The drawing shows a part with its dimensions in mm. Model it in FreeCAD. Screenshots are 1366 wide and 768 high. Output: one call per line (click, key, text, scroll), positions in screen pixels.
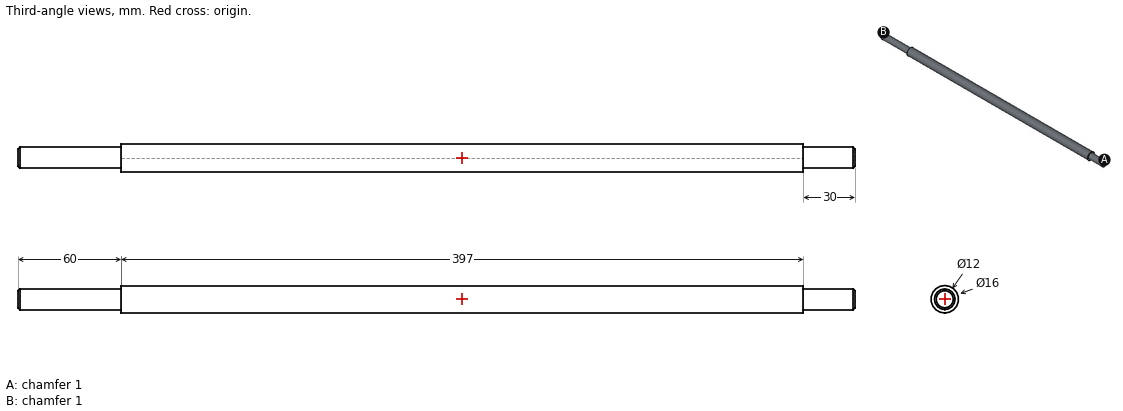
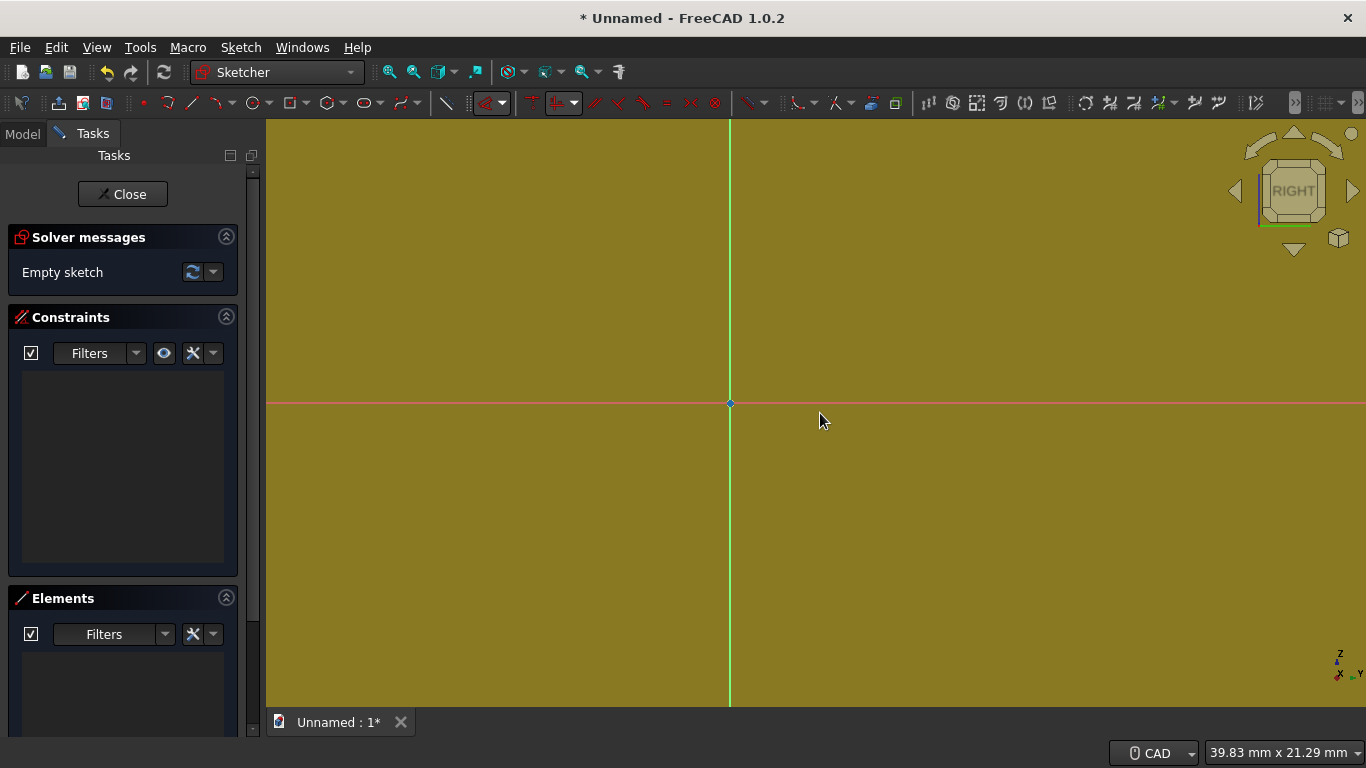
click(254, 104)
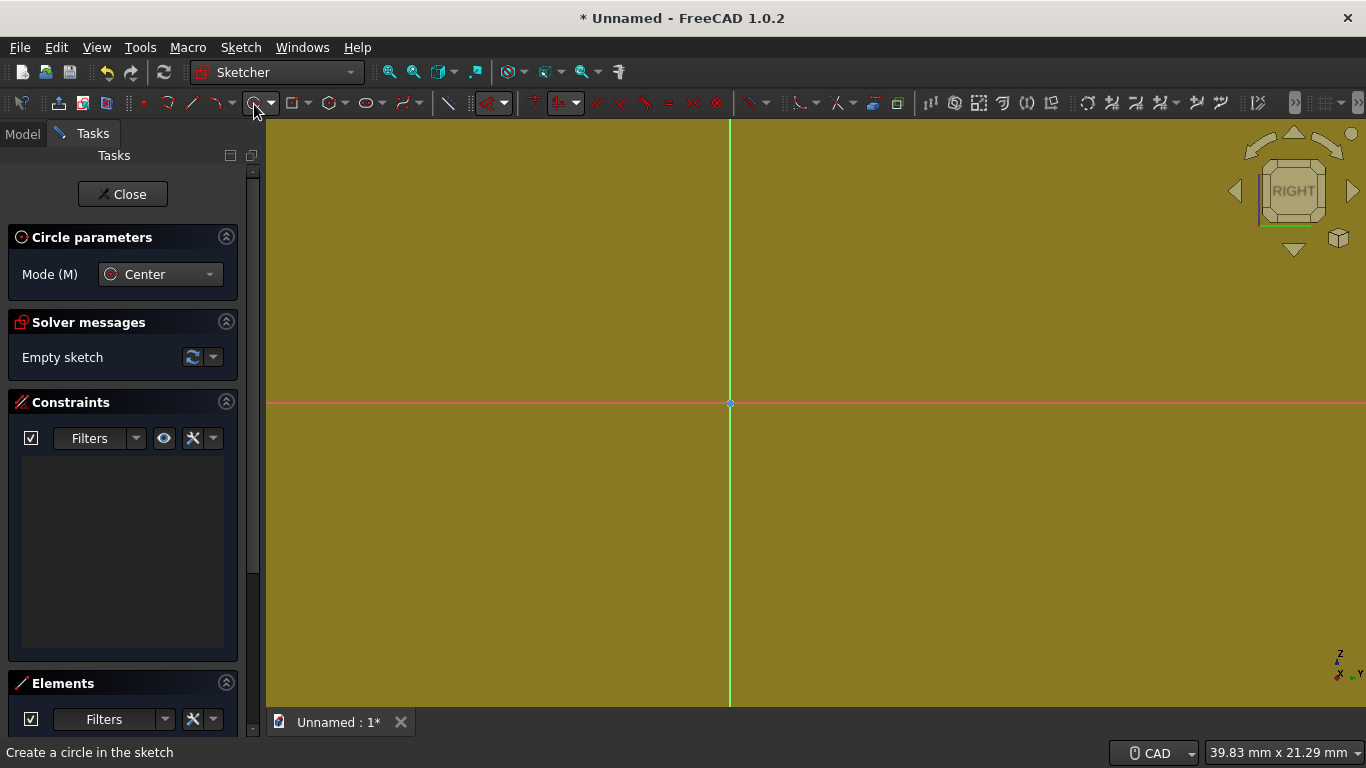
click(730, 403)
move(847, 286)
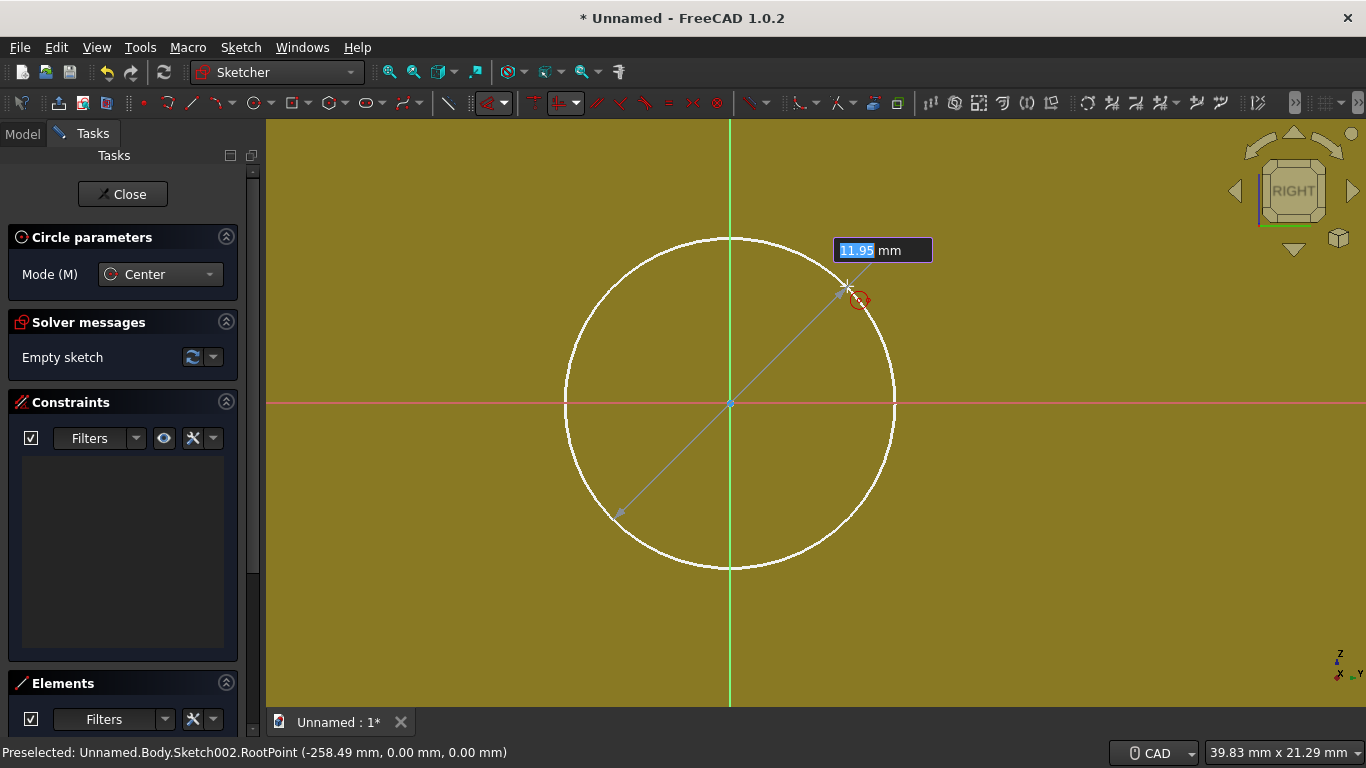
text(12)
key(Return)
key(Escape)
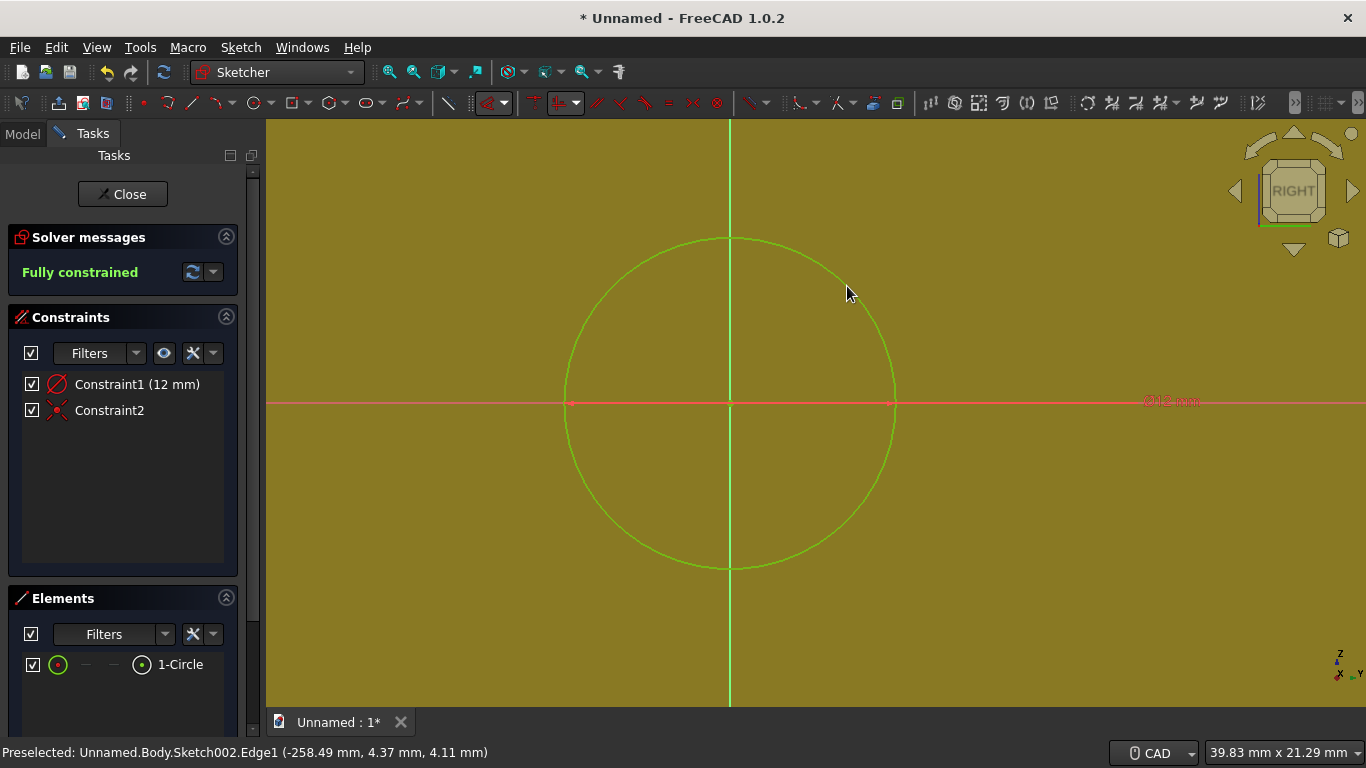
click(123, 194)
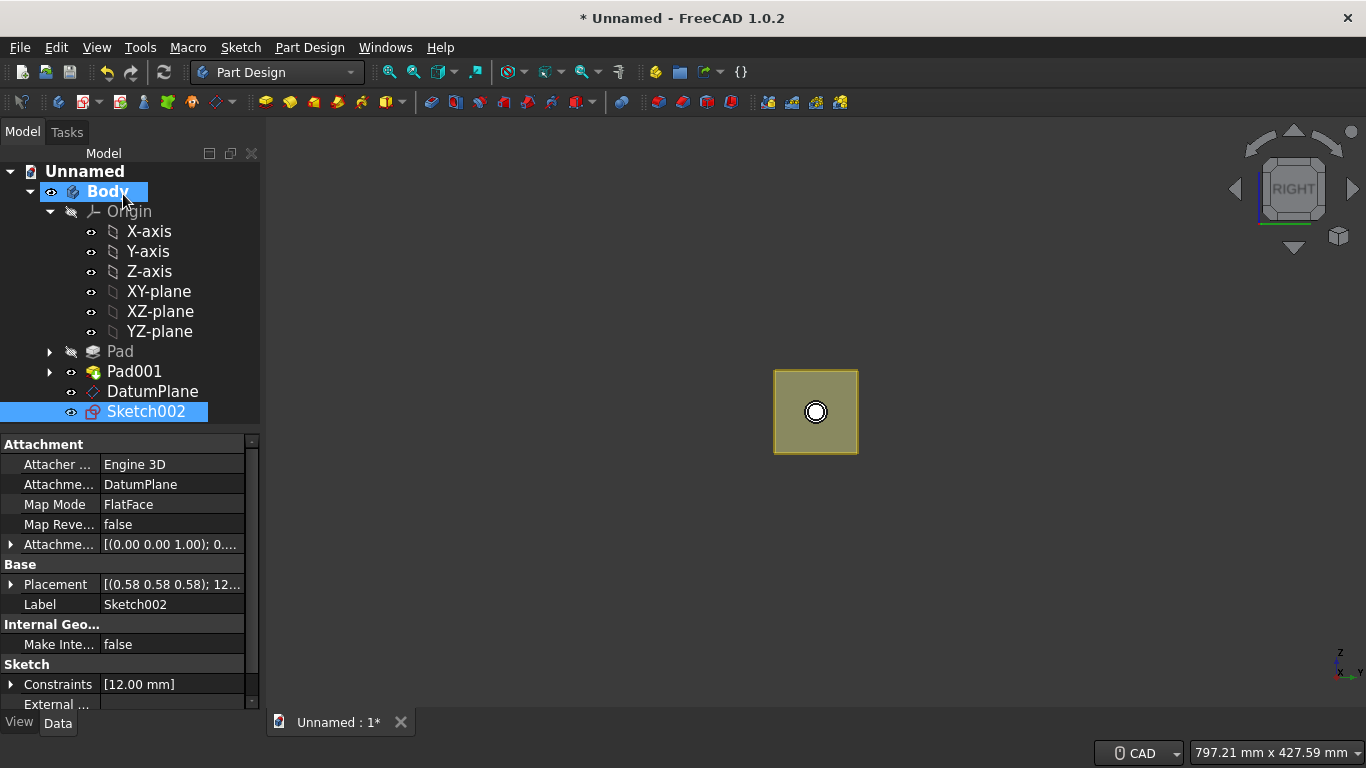
click(266, 102)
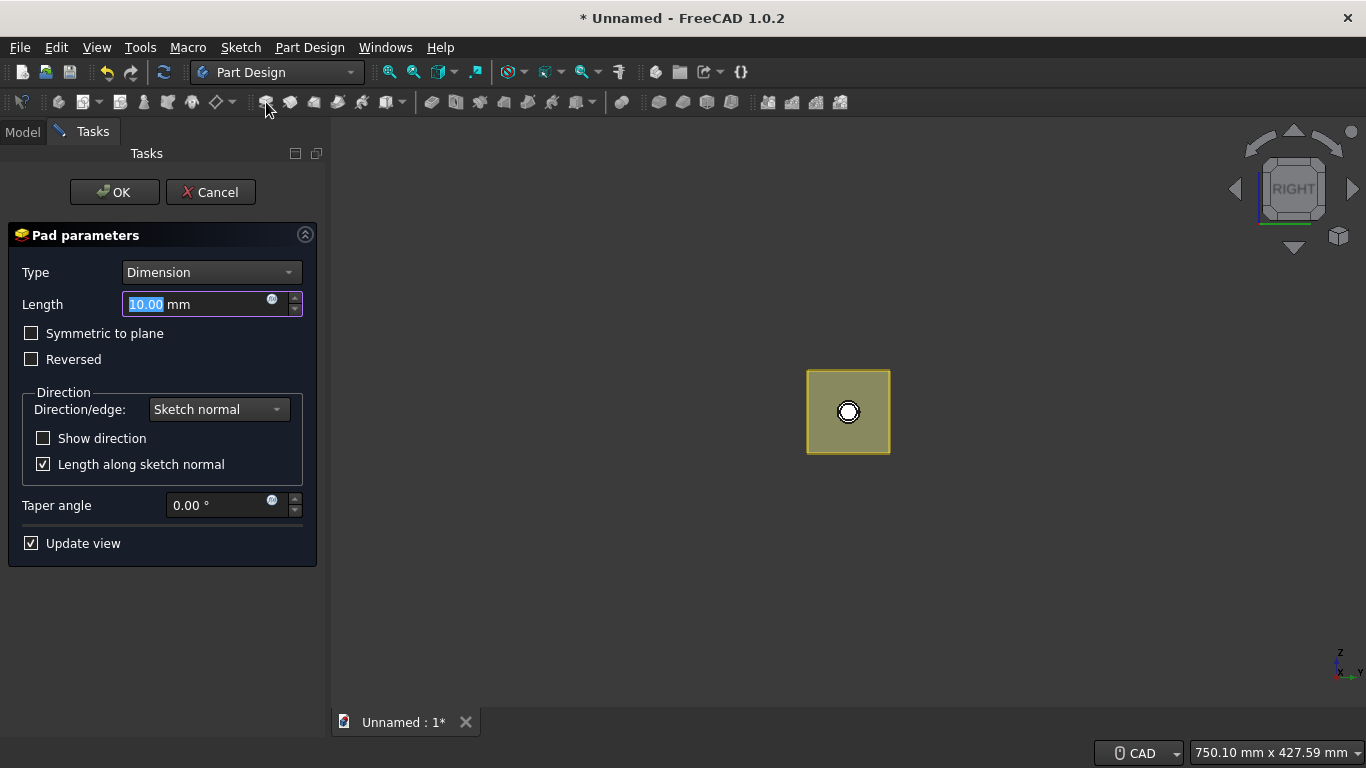
text(60)
key(Tab)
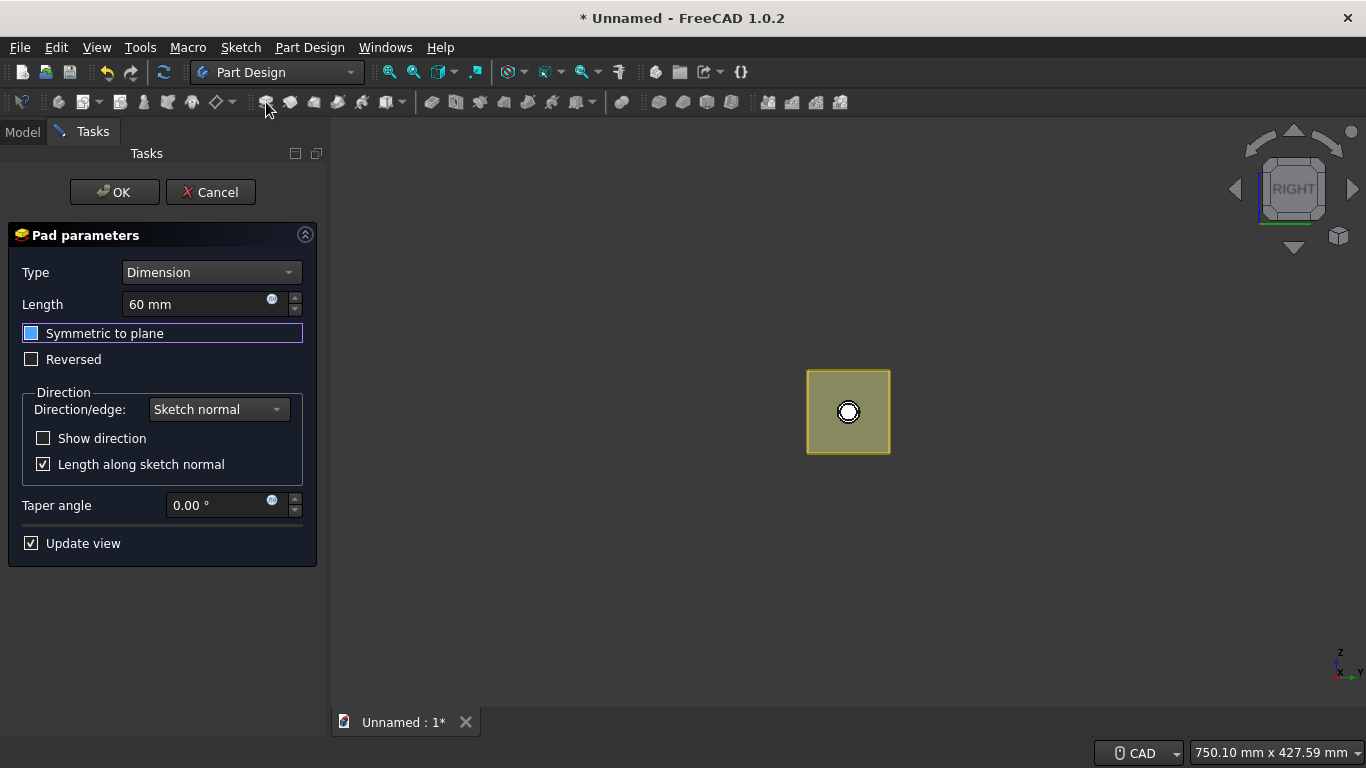
click(115, 192)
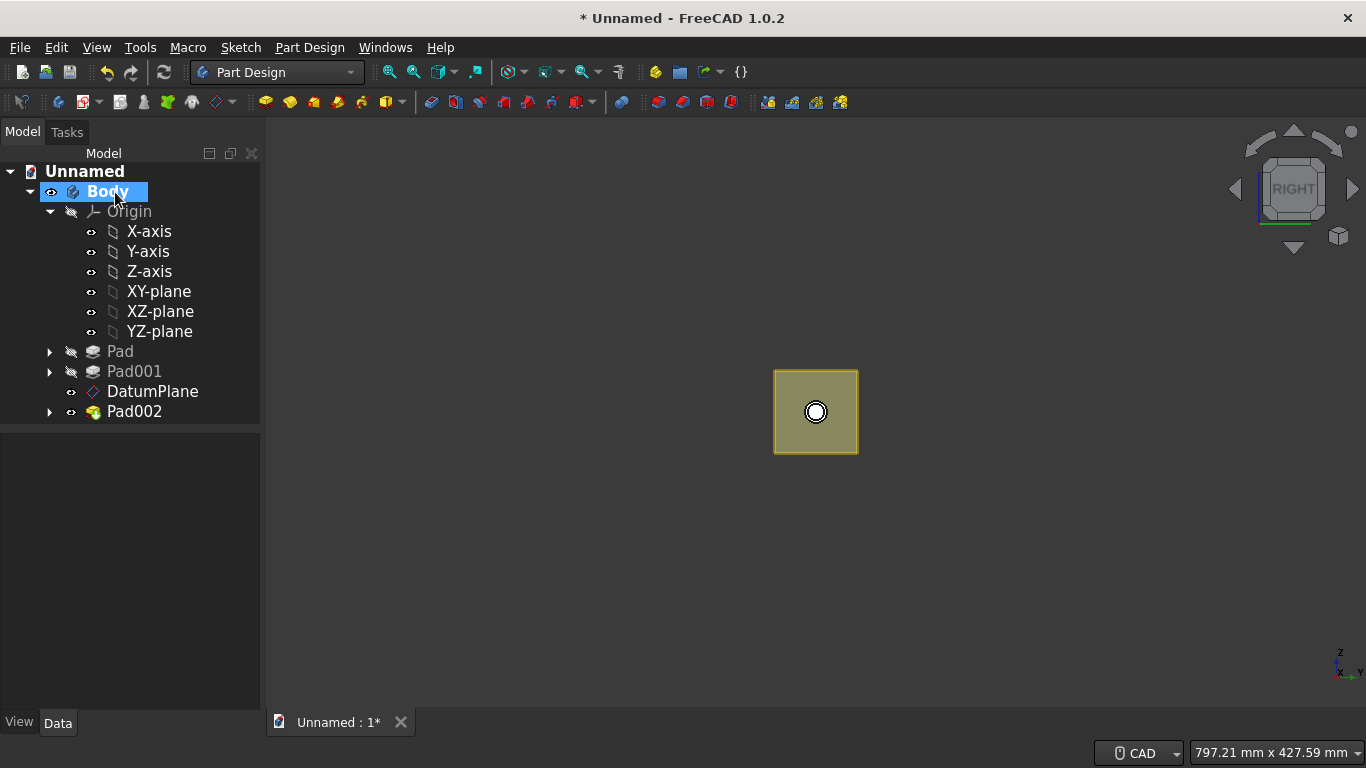
click(116, 392)
key(space)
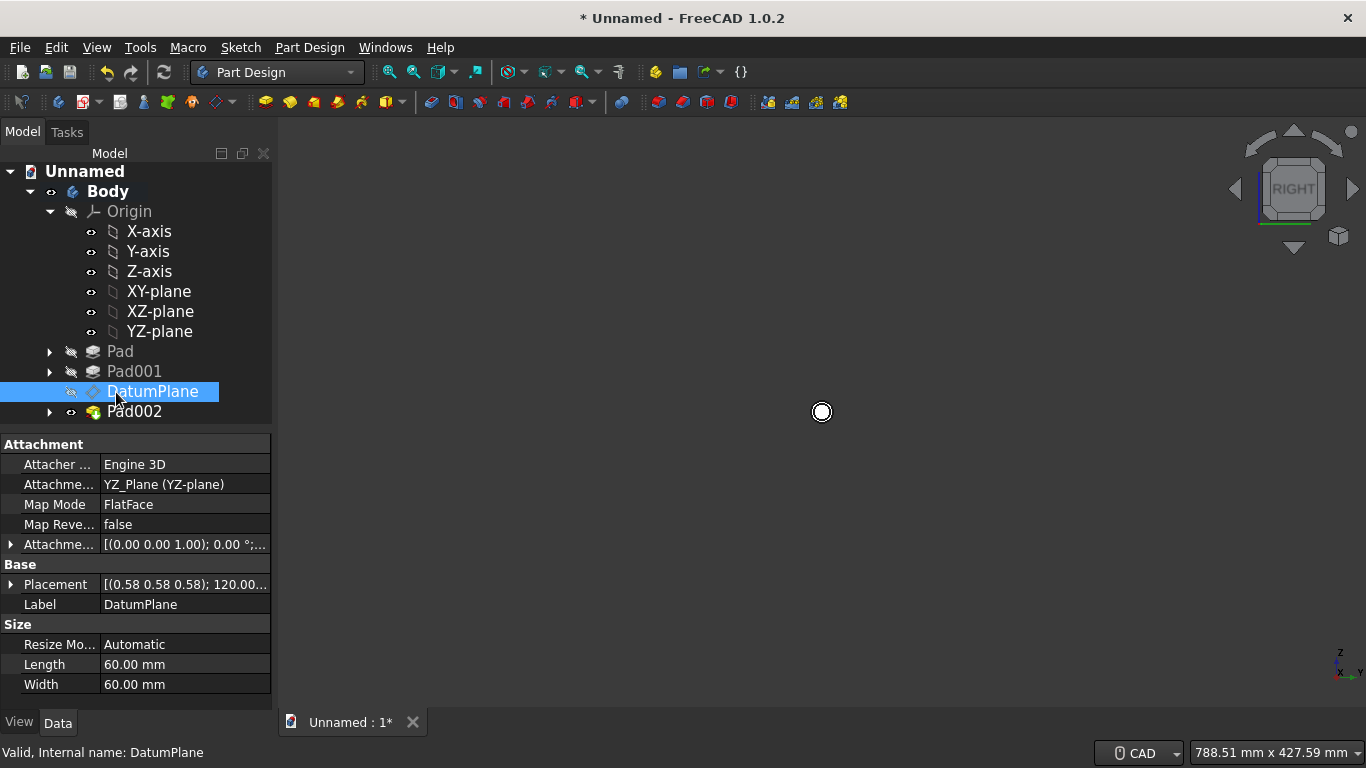
click(390, 72)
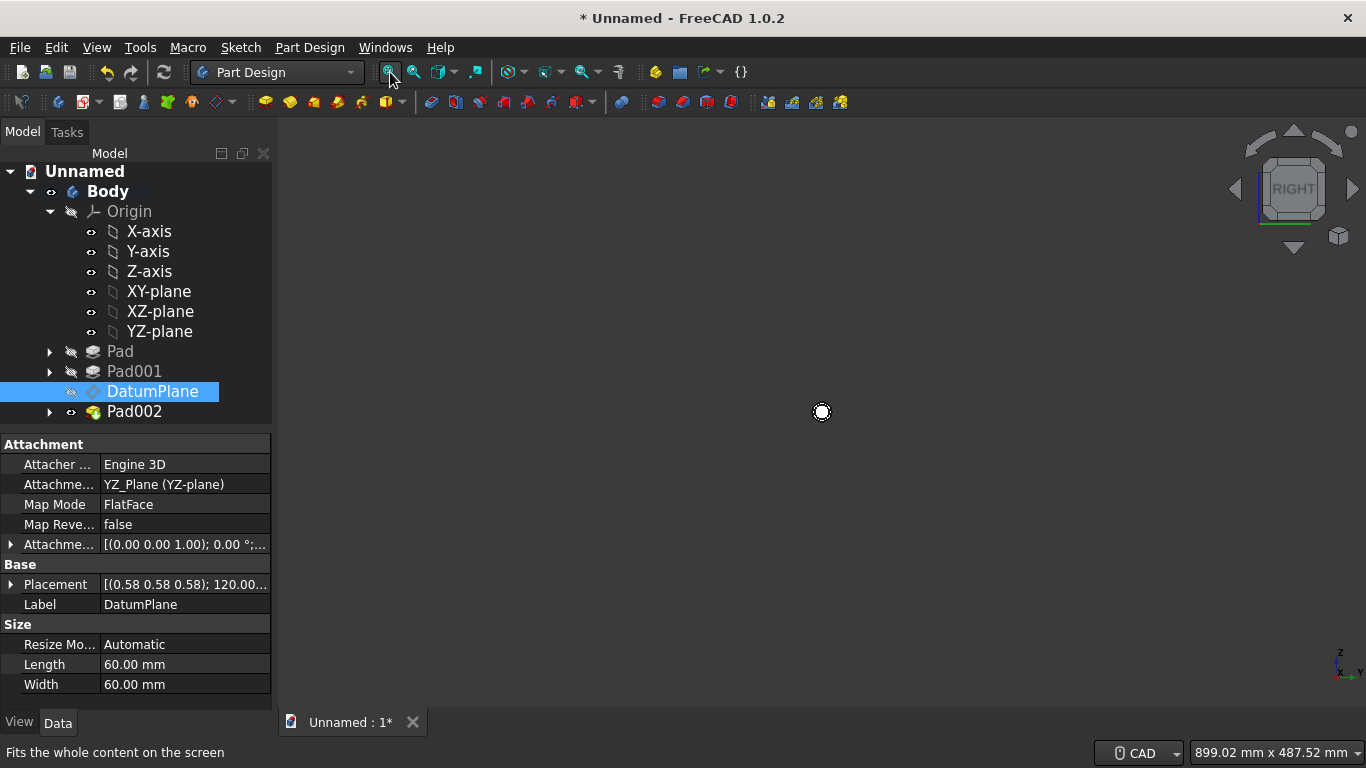
click(815, 411)